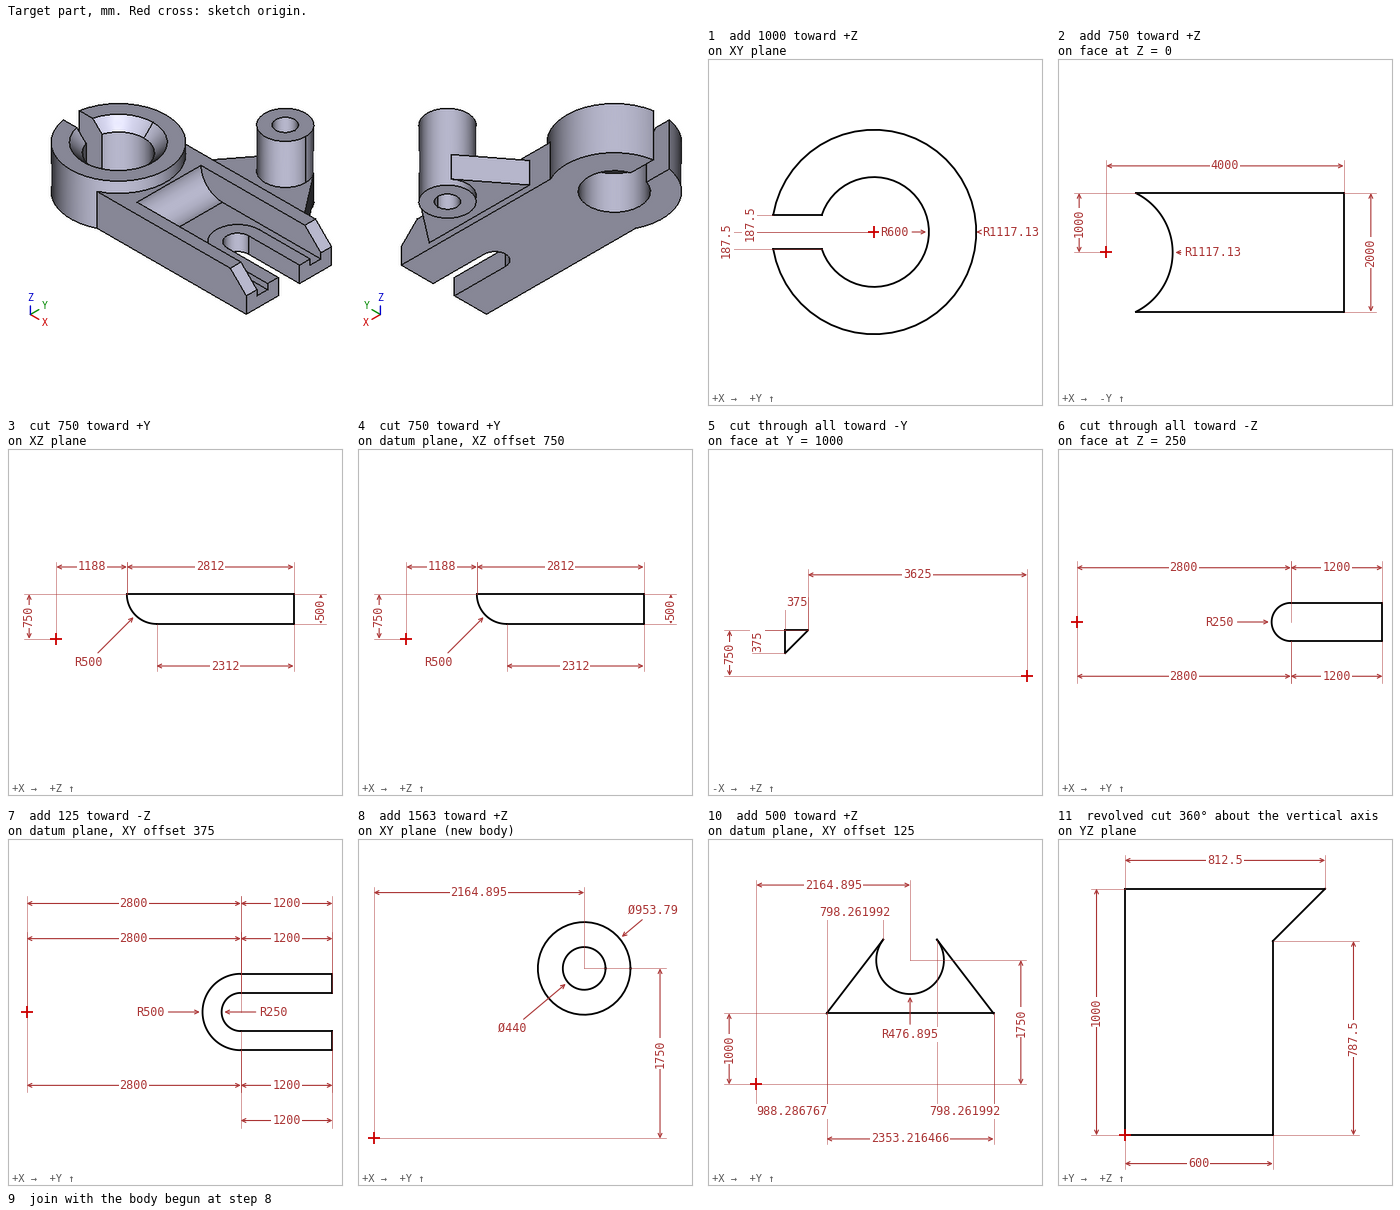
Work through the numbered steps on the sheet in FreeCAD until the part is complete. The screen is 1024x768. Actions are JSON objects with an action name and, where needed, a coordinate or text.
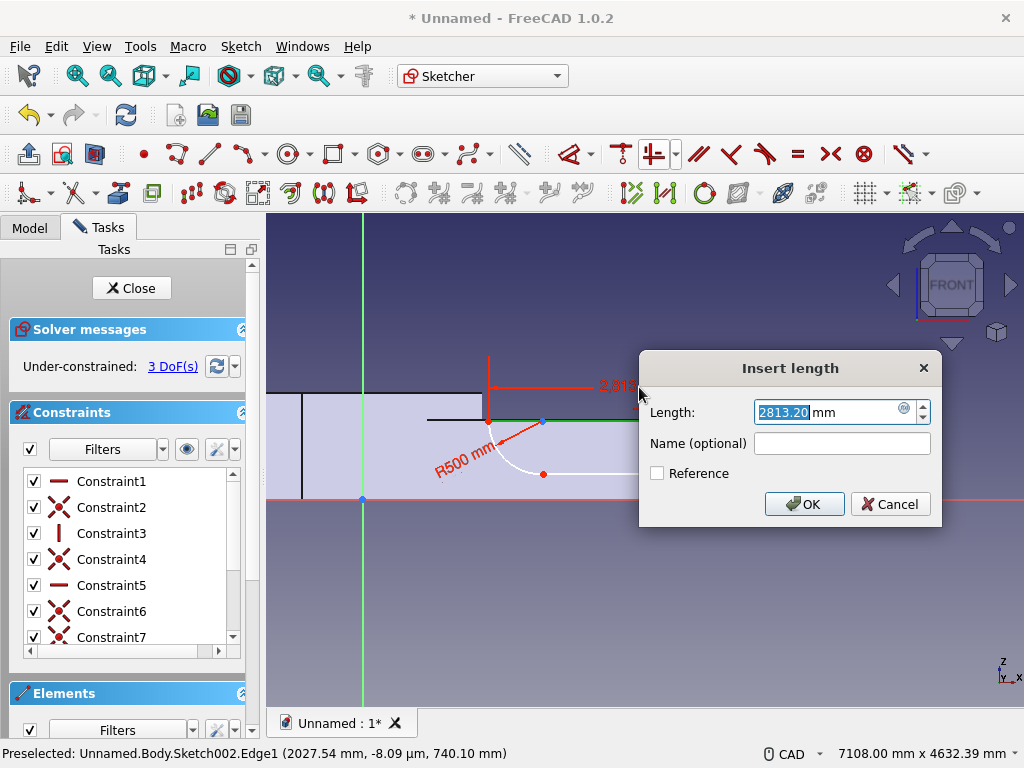
{"action": "type", "text": "2812"}
{"action": "key", "text": "Return"}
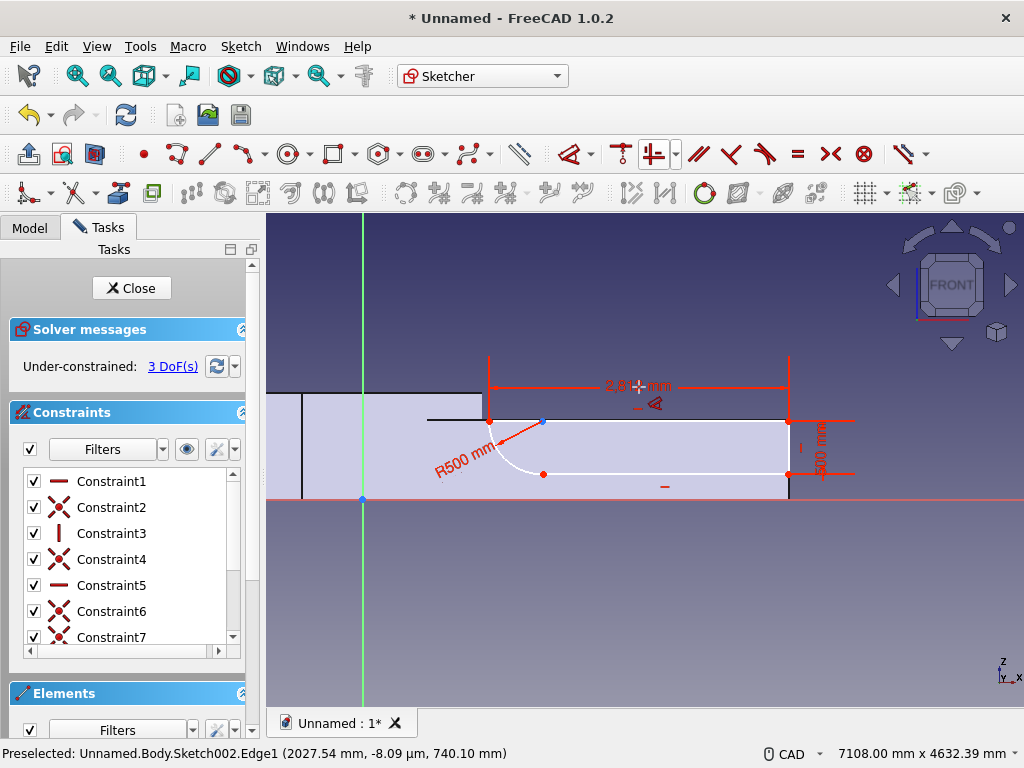
{"action": "left_click", "coordinate": [715, 474]}
{"action": "left_click", "coordinate": [666, 440]}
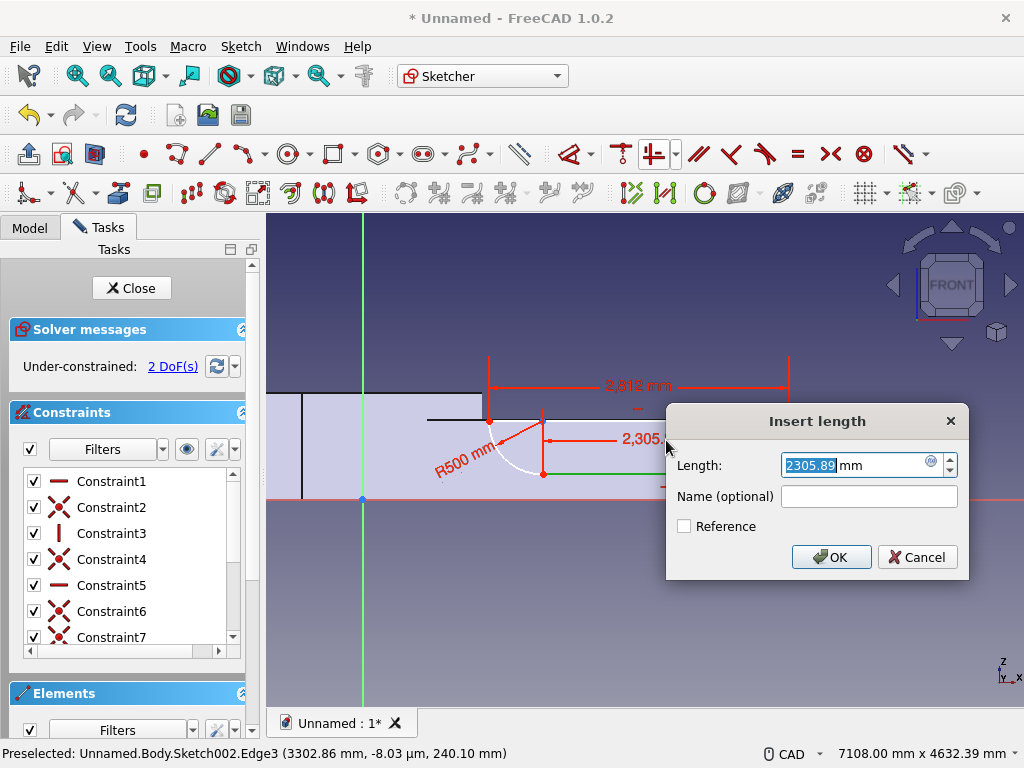
{"action": "type", "text": "2312"}
{"action": "key", "text": "Return"}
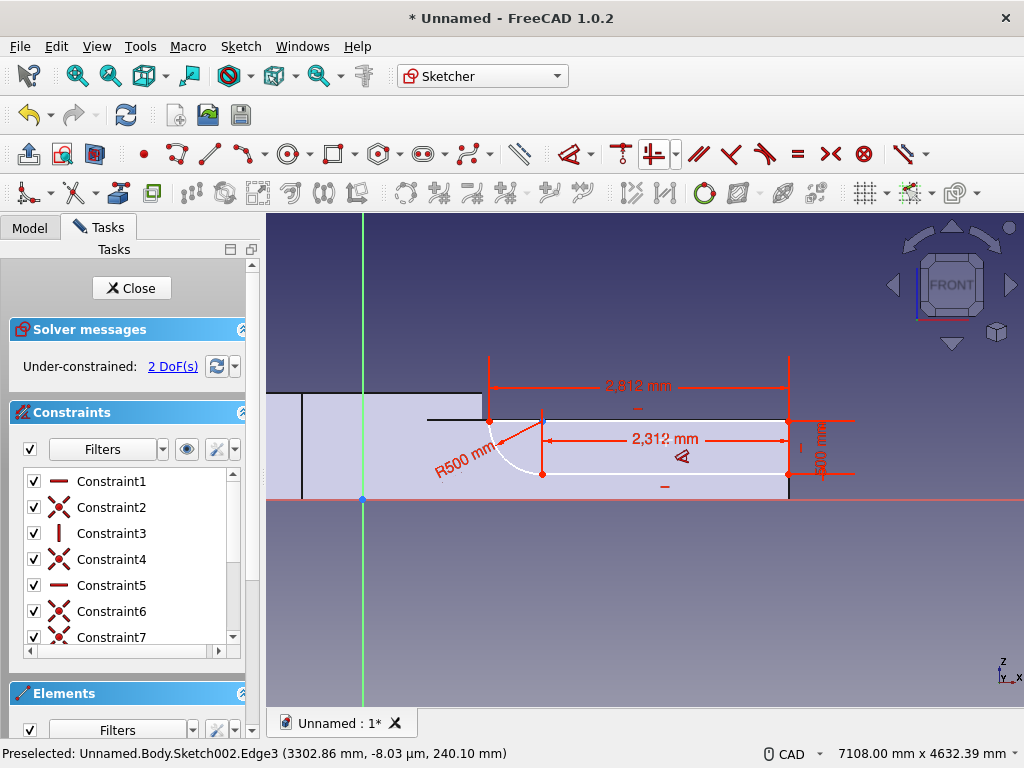
{"action": "left_click", "coordinate": [489, 421]}
{"action": "left_click", "coordinate": [329, 460]}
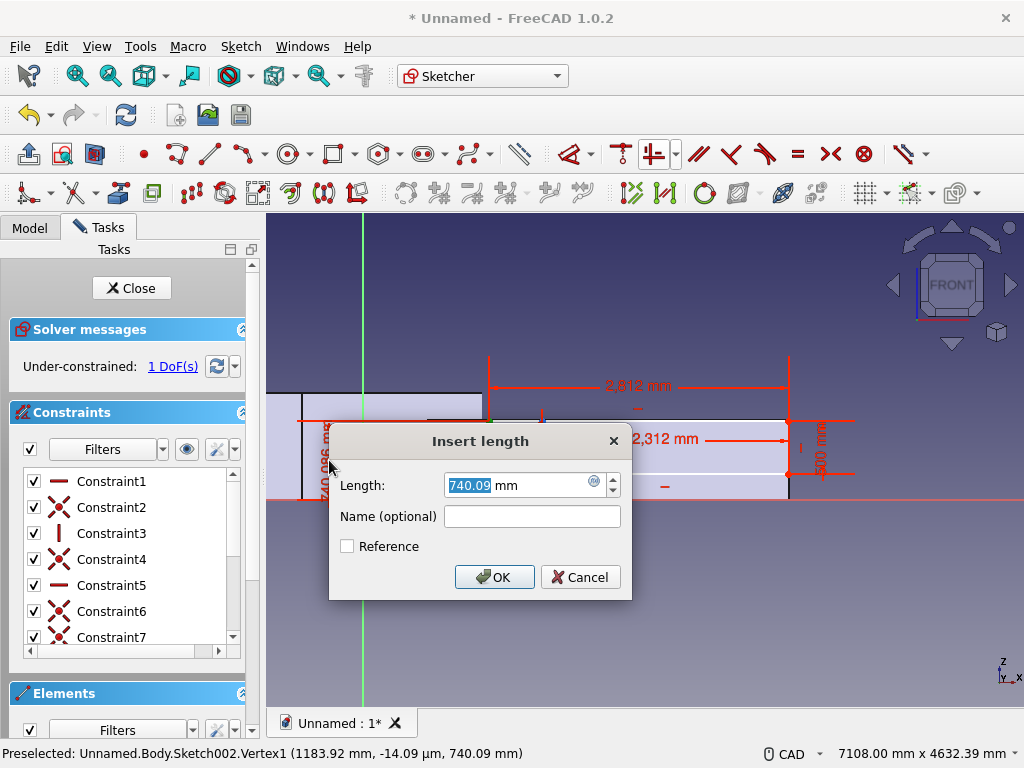
{"action": "type", "text": "750"}
{"action": "key", "text": "Return"}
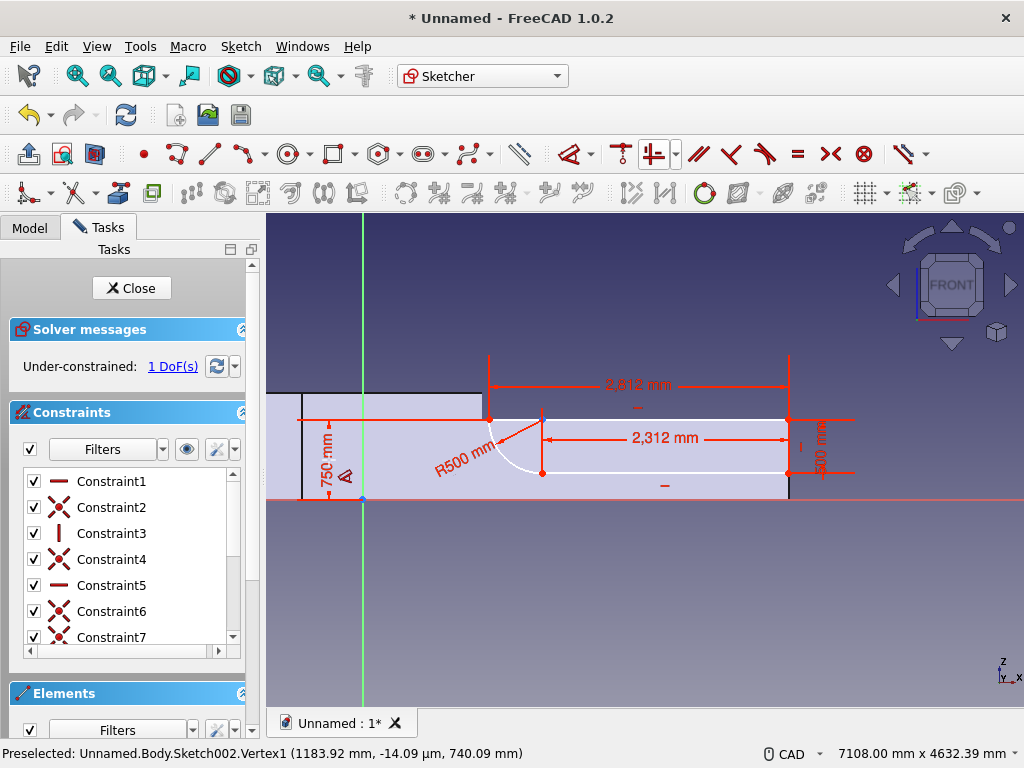
{"action": "left_click", "coordinate": [489, 420]}
{"action": "left_click", "coordinate": [426, 534]}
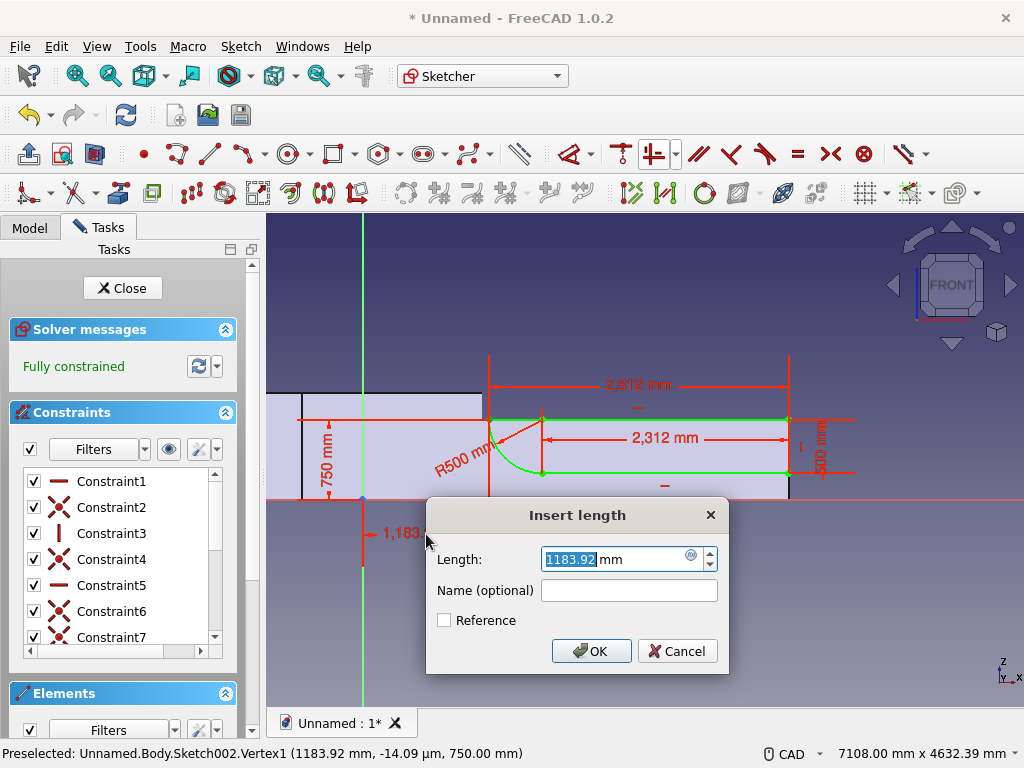
{"action": "type", "text": "1188"}
{"action": "key", "text": "Return"}
{"action": "key", "text": "Escape"}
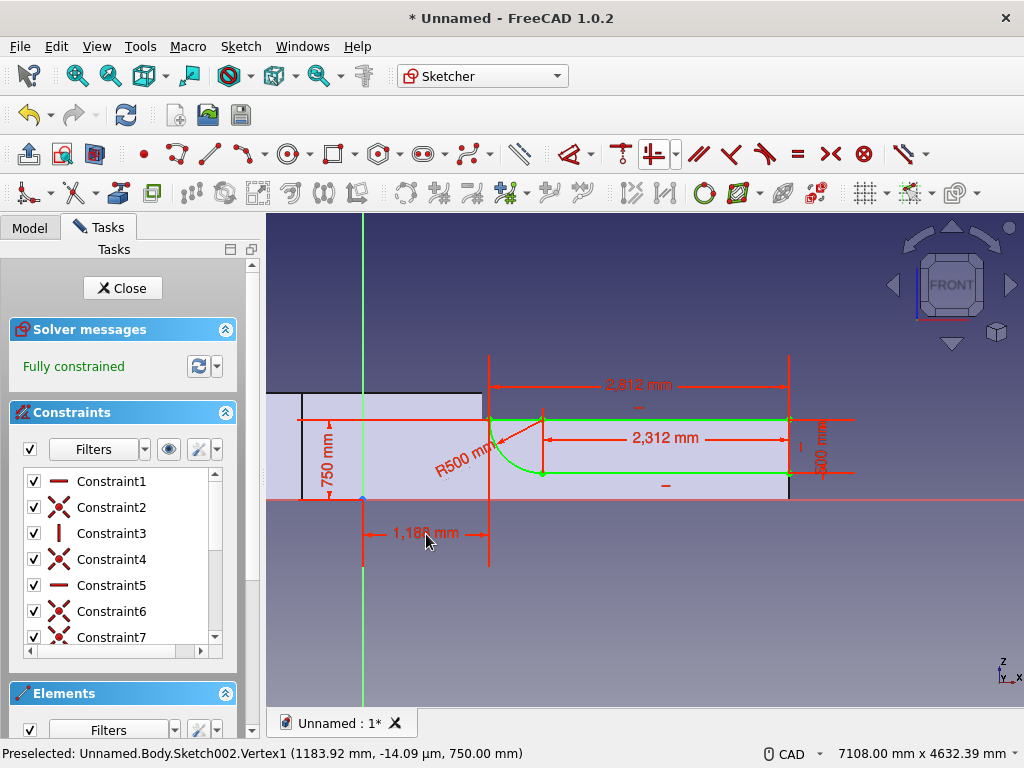
{"action": "left_click", "coordinate": [123, 288]}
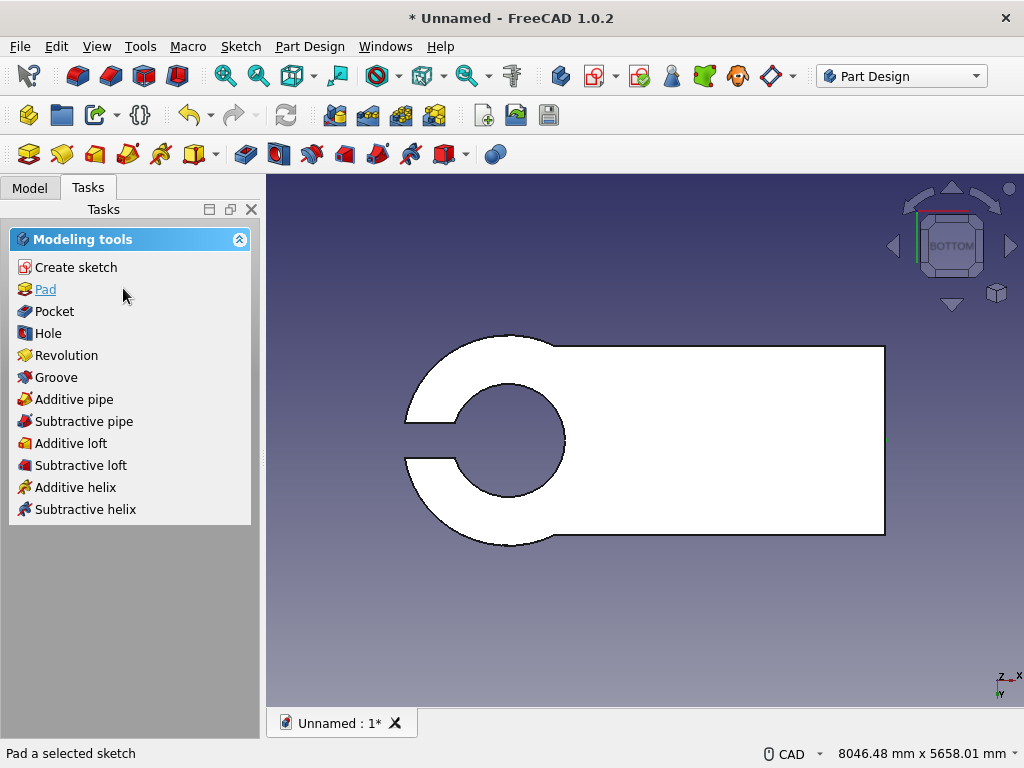
{"action": "left_click", "coordinate": [246, 154]}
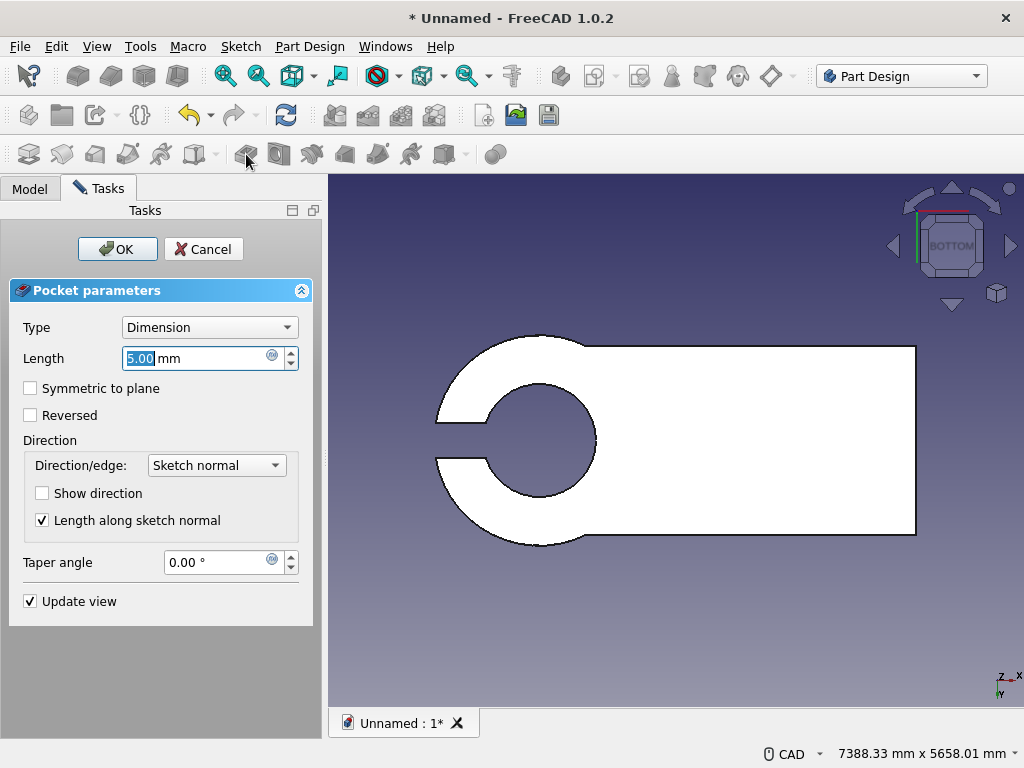
{"action": "type", "text": "750"}
{"action": "key", "text": "Tab"}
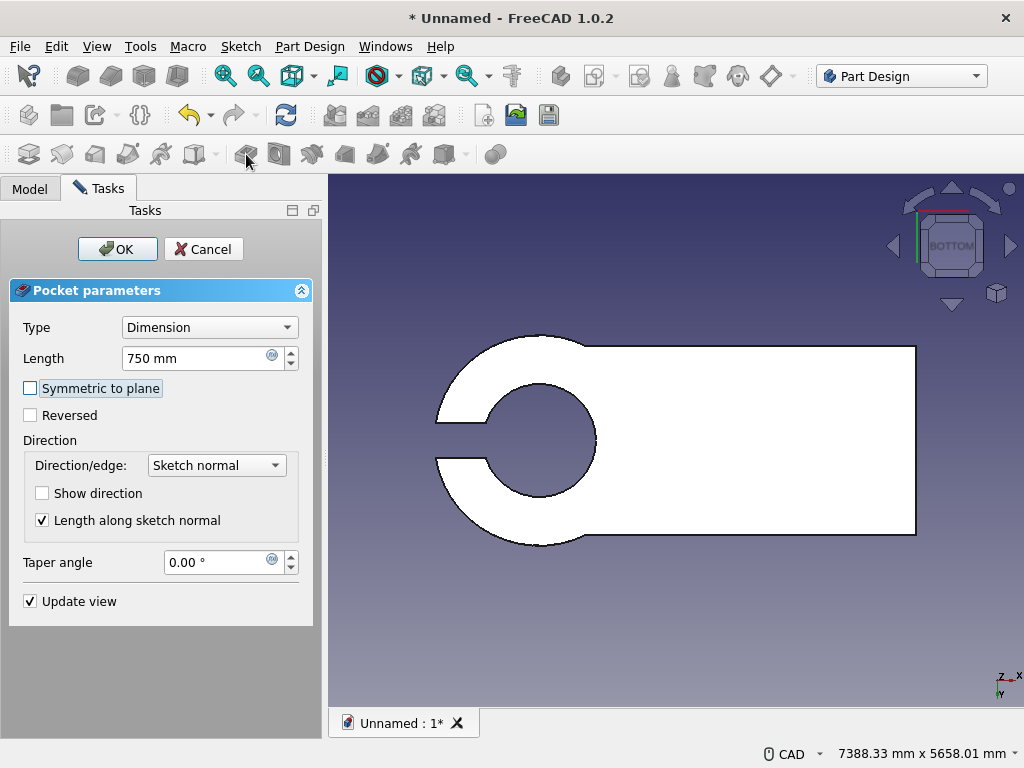
{"action": "left_click", "coordinate": [118, 249]}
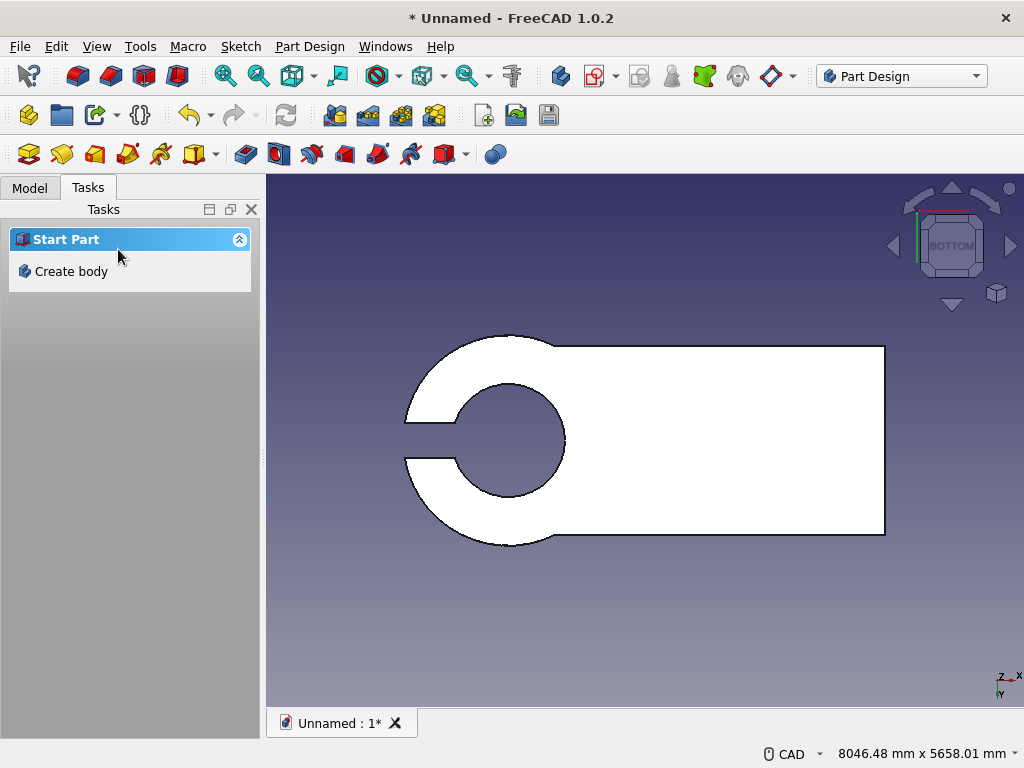
{"action": "left_click", "coordinate": [30, 188]}